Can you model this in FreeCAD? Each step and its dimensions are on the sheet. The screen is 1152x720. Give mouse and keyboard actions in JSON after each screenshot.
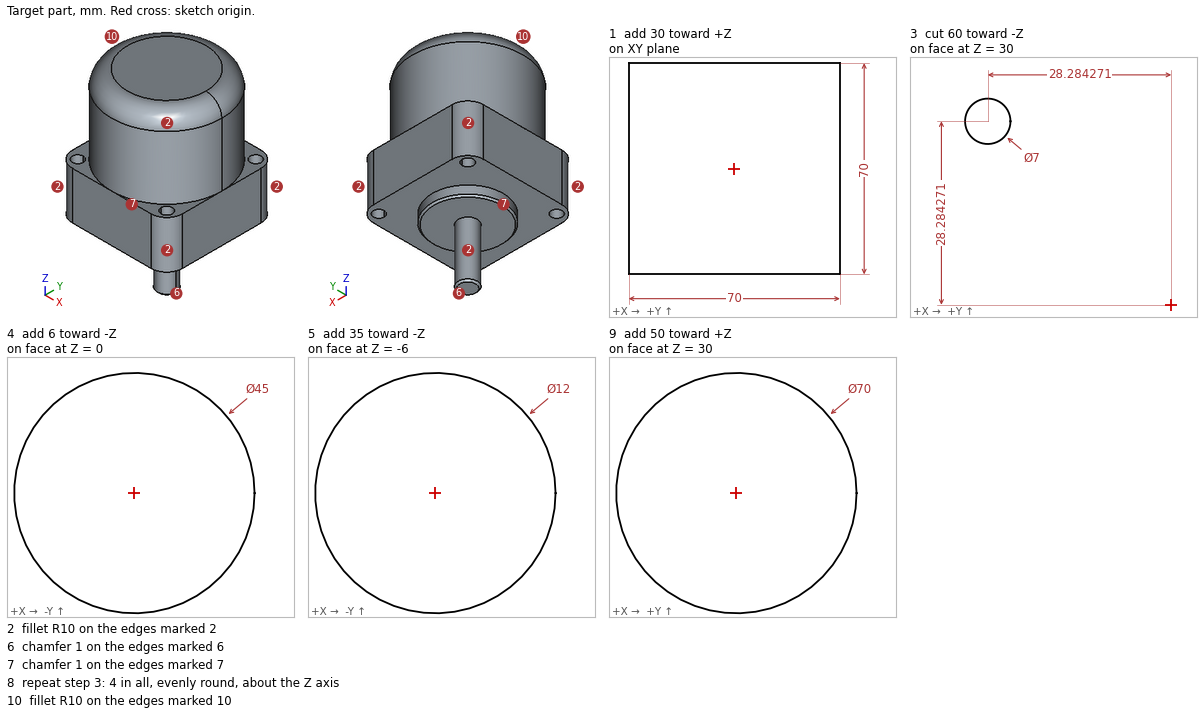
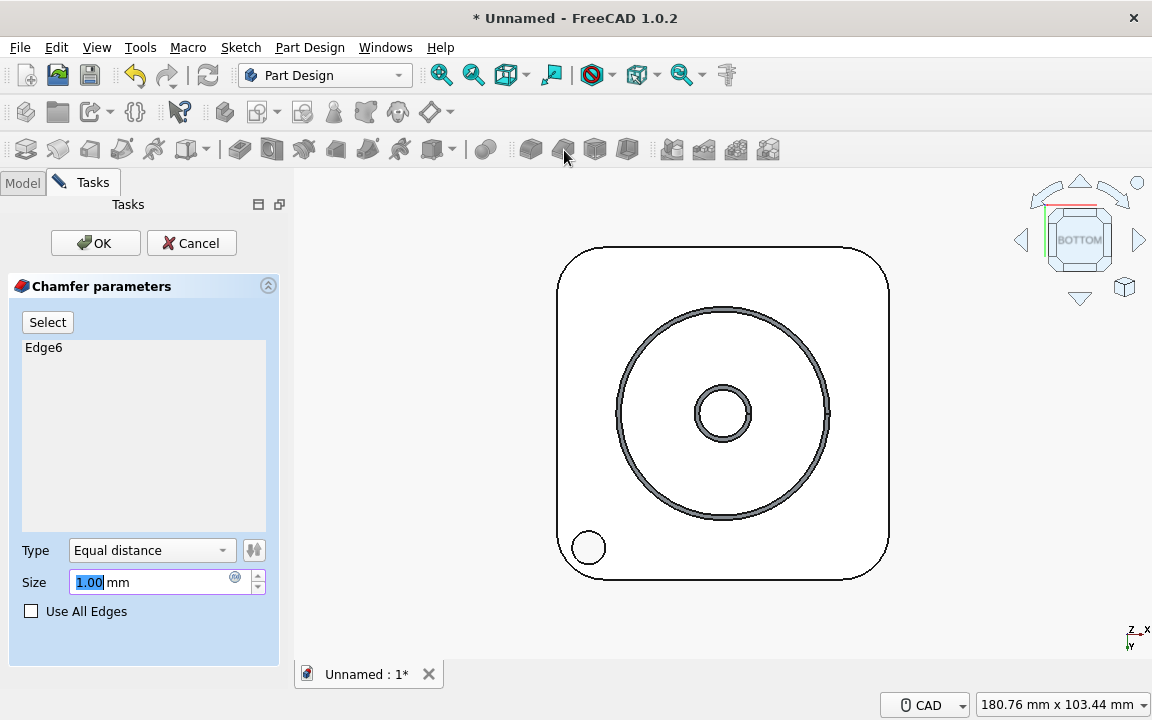
{"action": "type", "text": "1"}
{"action": "key", "text": "Tab"}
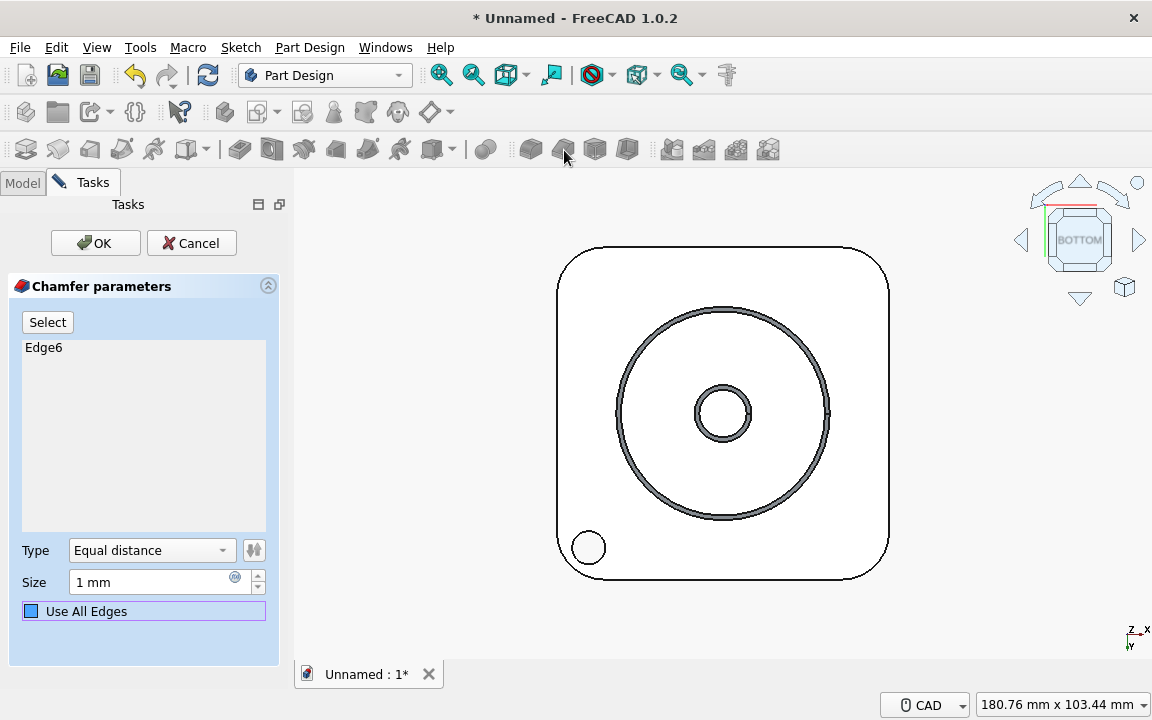
{"action": "left_click", "coordinate": [96, 243]}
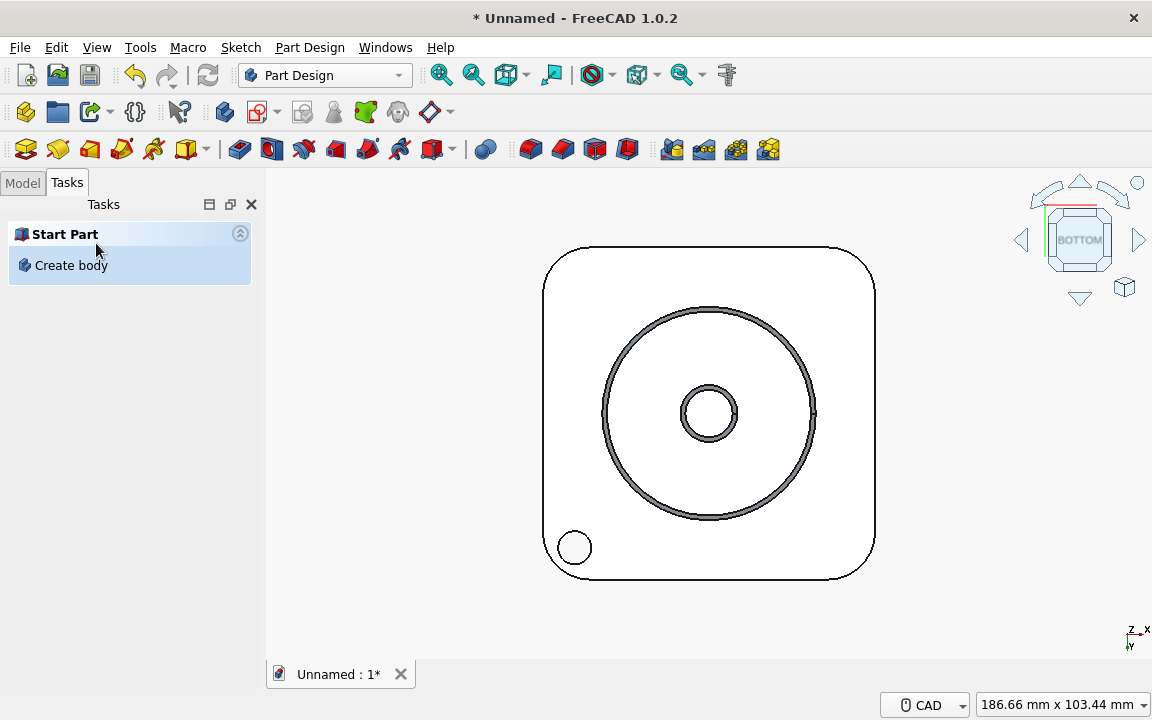
{"action": "left_click", "coordinate": [23, 182]}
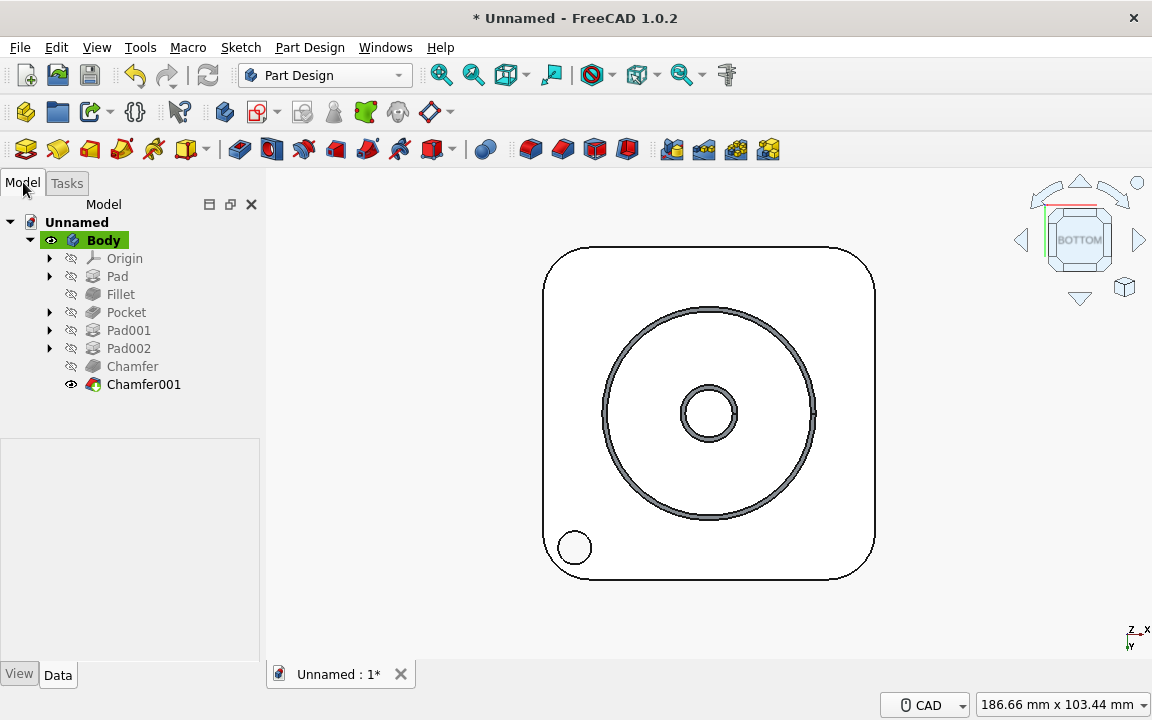
{"action": "left_click", "coordinate": [116, 312]}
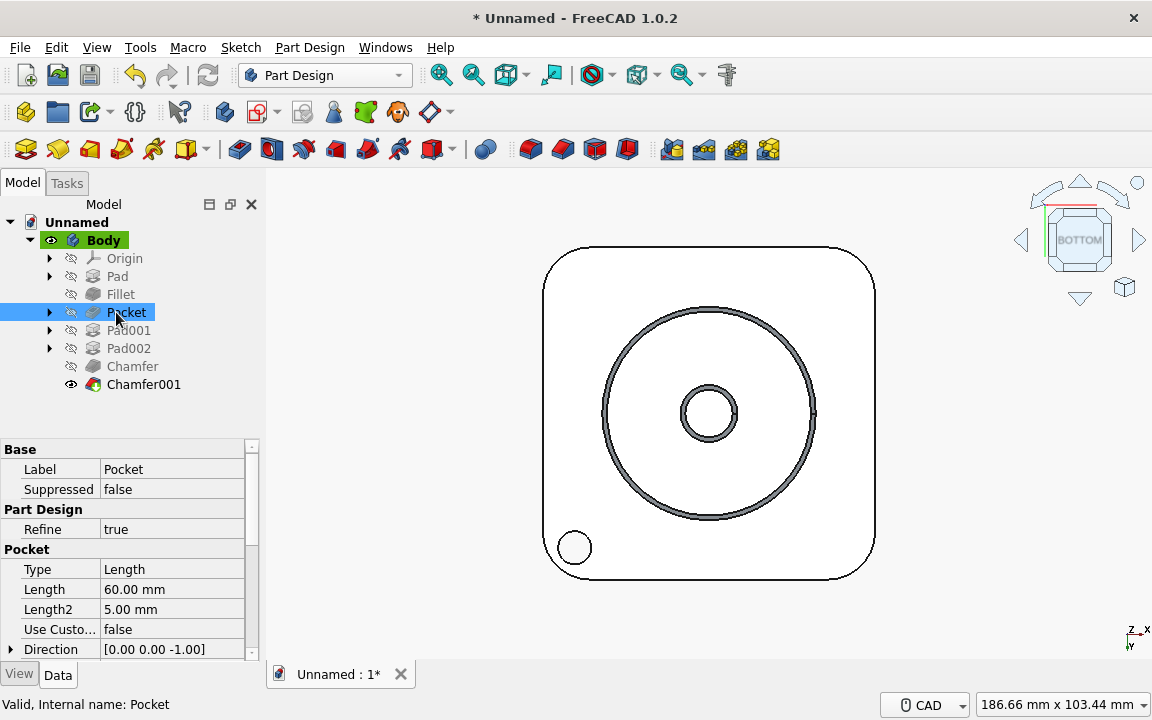
{"action": "left_click", "coordinate": [736, 150]}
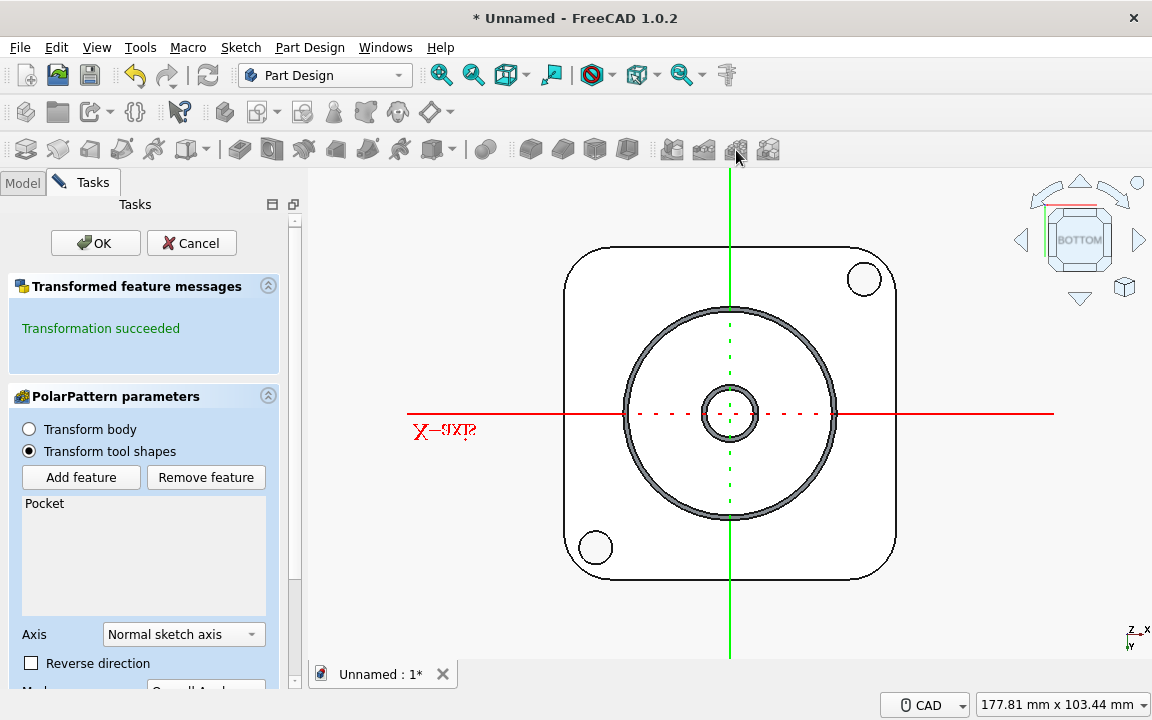
{"action": "left_click", "coordinate": [184, 634]}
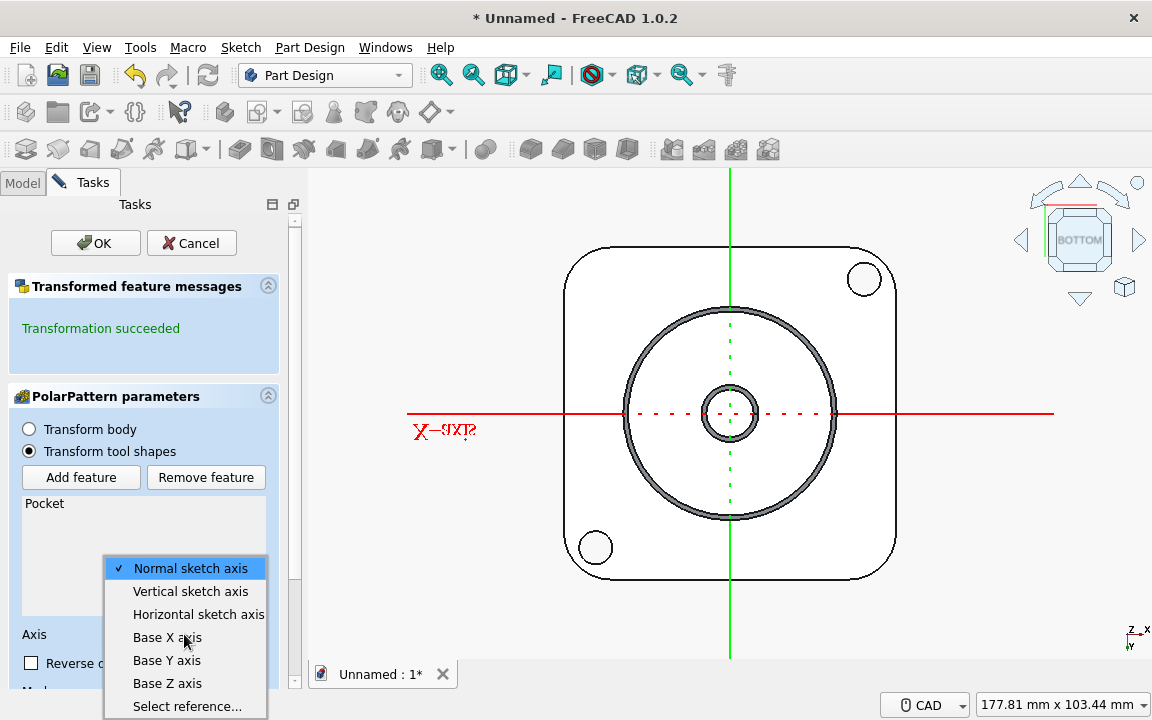
{"action": "left_click", "coordinate": [184, 684]}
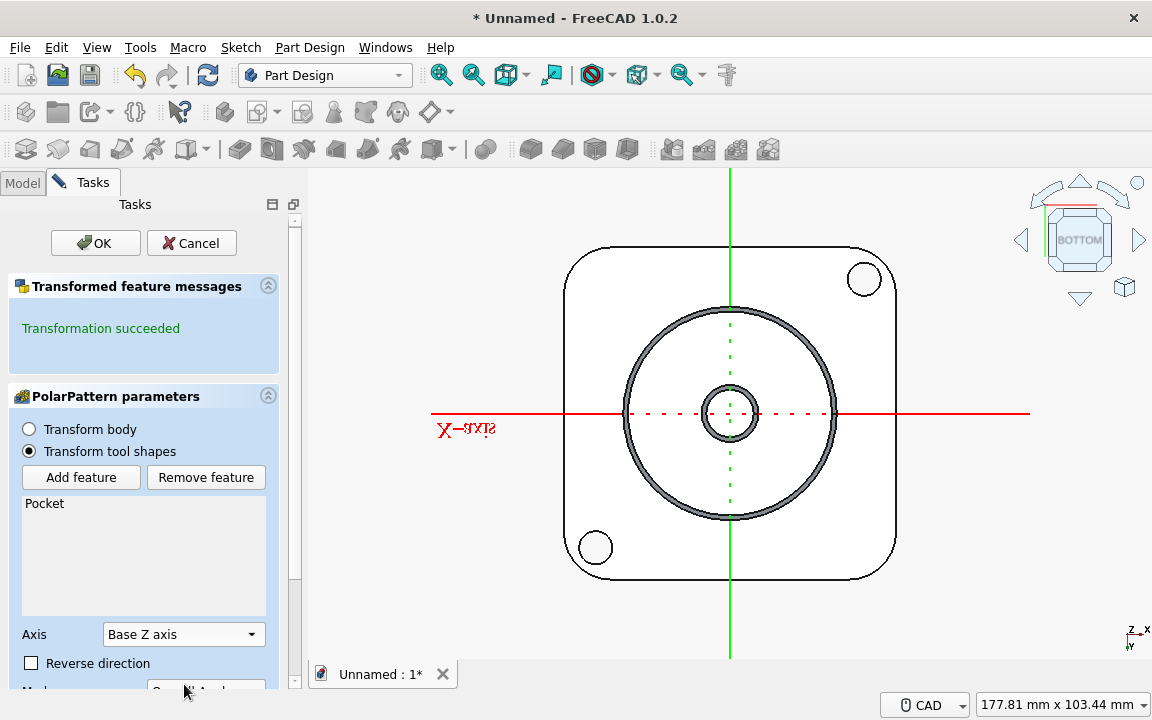
{"action": "scroll", "coordinate": [295, 451], "scroll_direction": "down", "scroll_amount": 3}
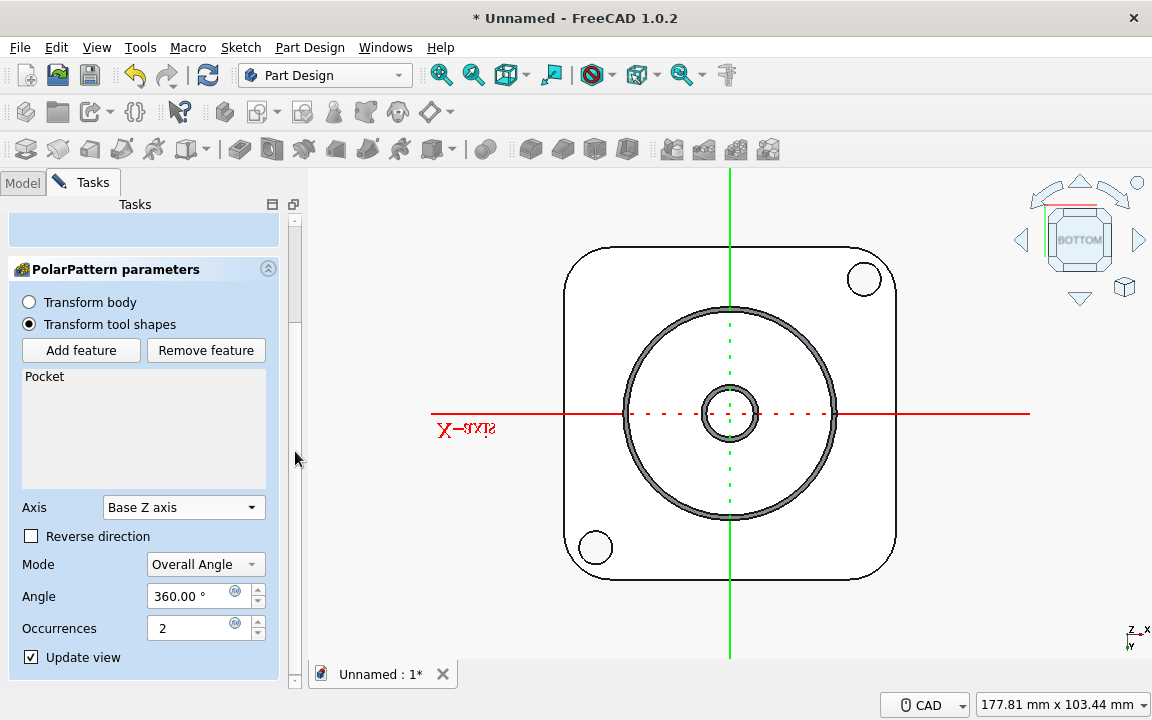
{"action": "triple_click", "coordinate": [198, 628]}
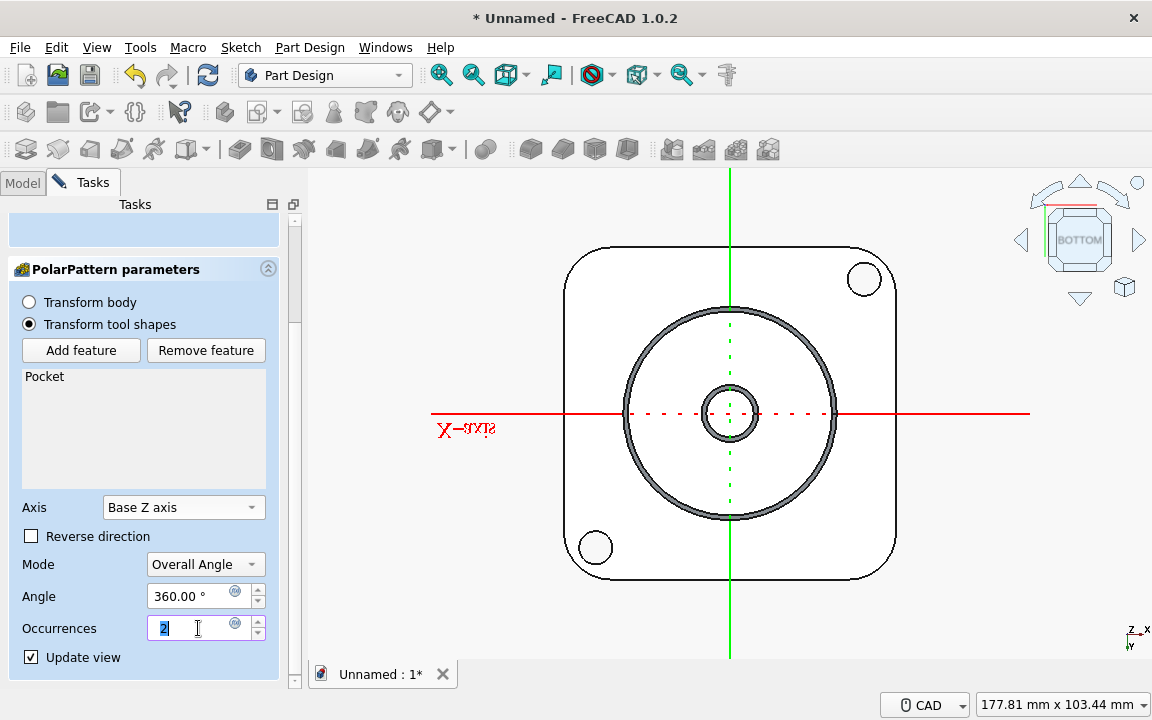
{"action": "type", "text": "4"}
{"action": "key", "text": "Tab"}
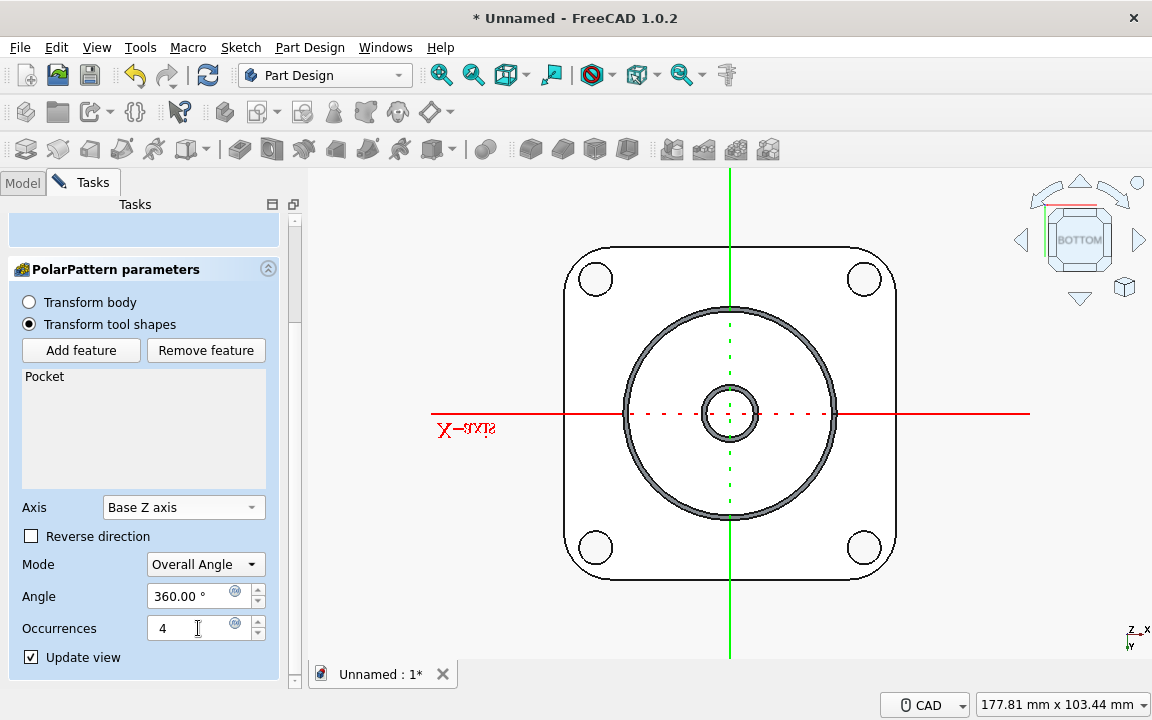
{"action": "scroll", "coordinate": [295, 451], "scroll_direction": "up", "scroll_amount": 3}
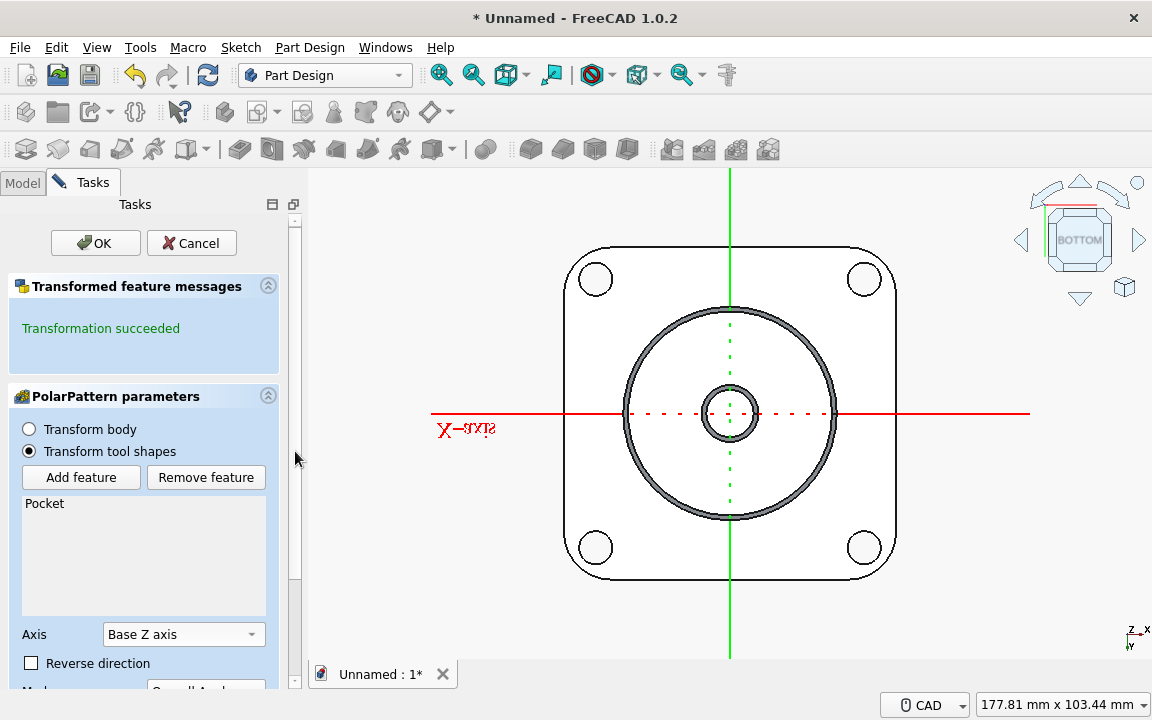
{"action": "left_click", "coordinate": [96, 243]}